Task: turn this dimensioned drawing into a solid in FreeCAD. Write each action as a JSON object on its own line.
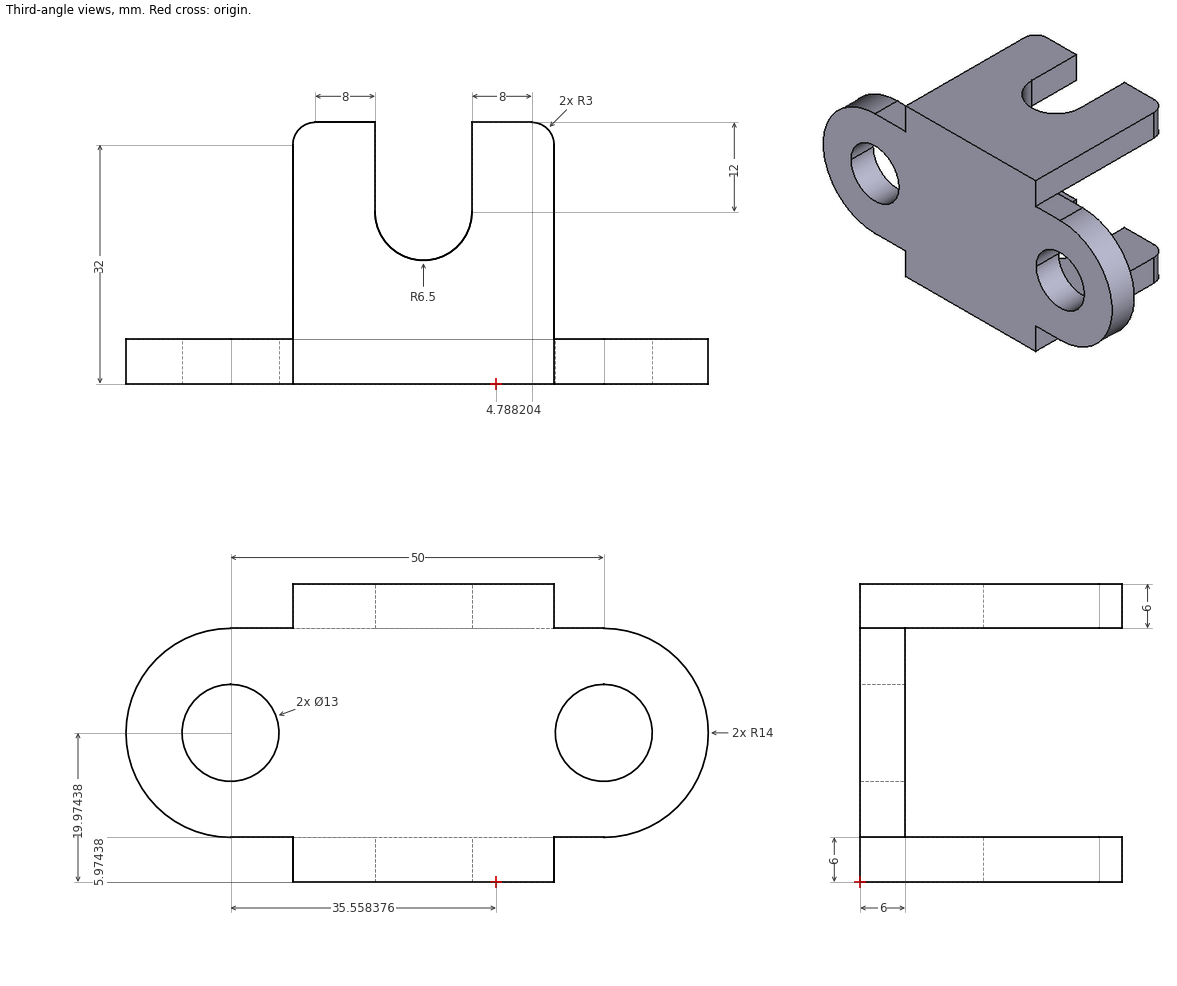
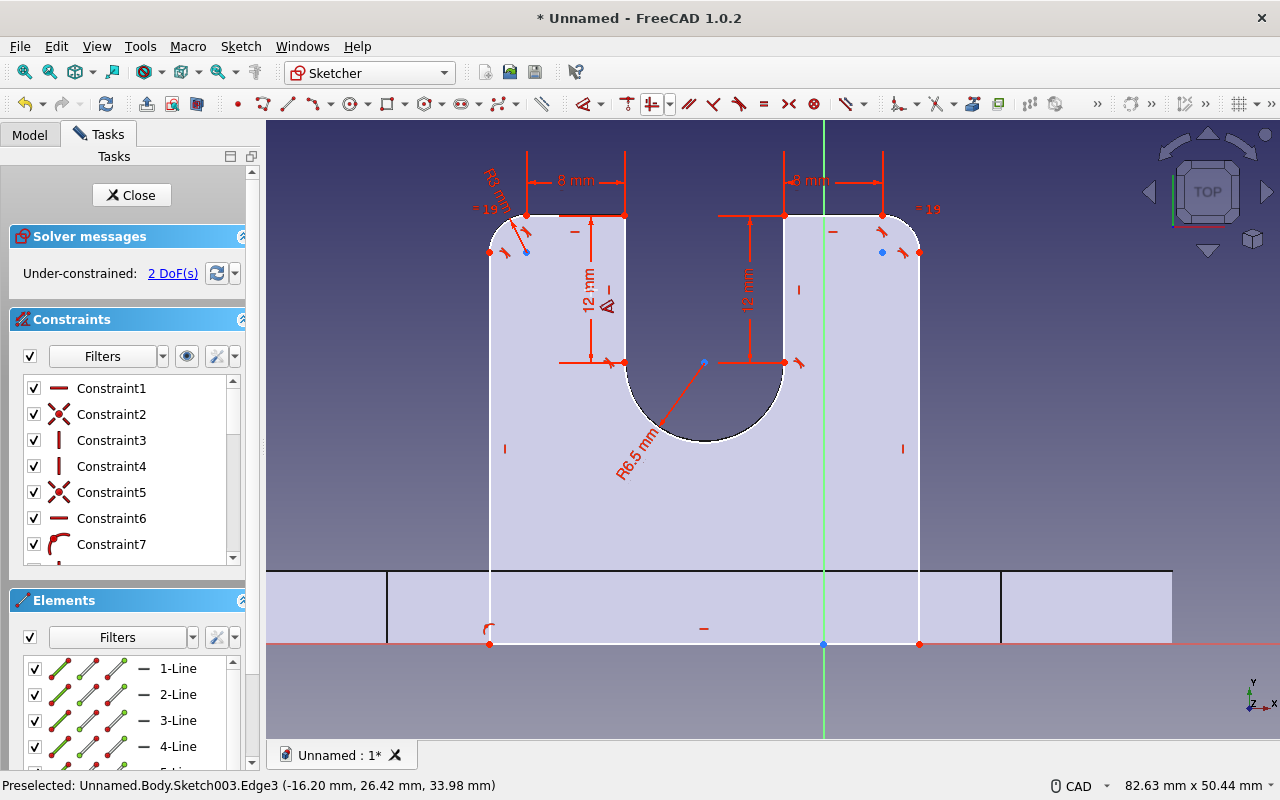
{"action": "left_click", "coordinate": [490, 370]}
{"action": "left_click", "coordinate": [456, 448]}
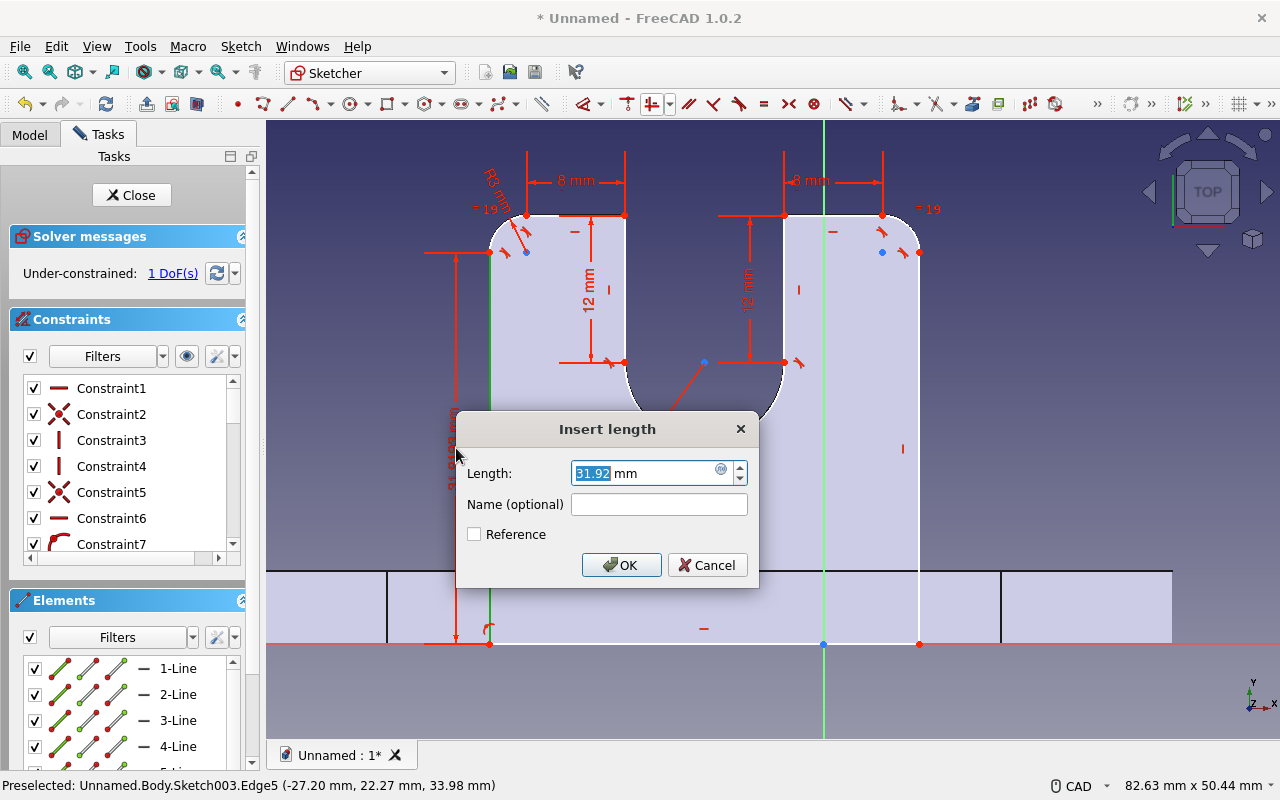
{"action": "type", "text": "32"}
{"action": "key", "text": "Return"}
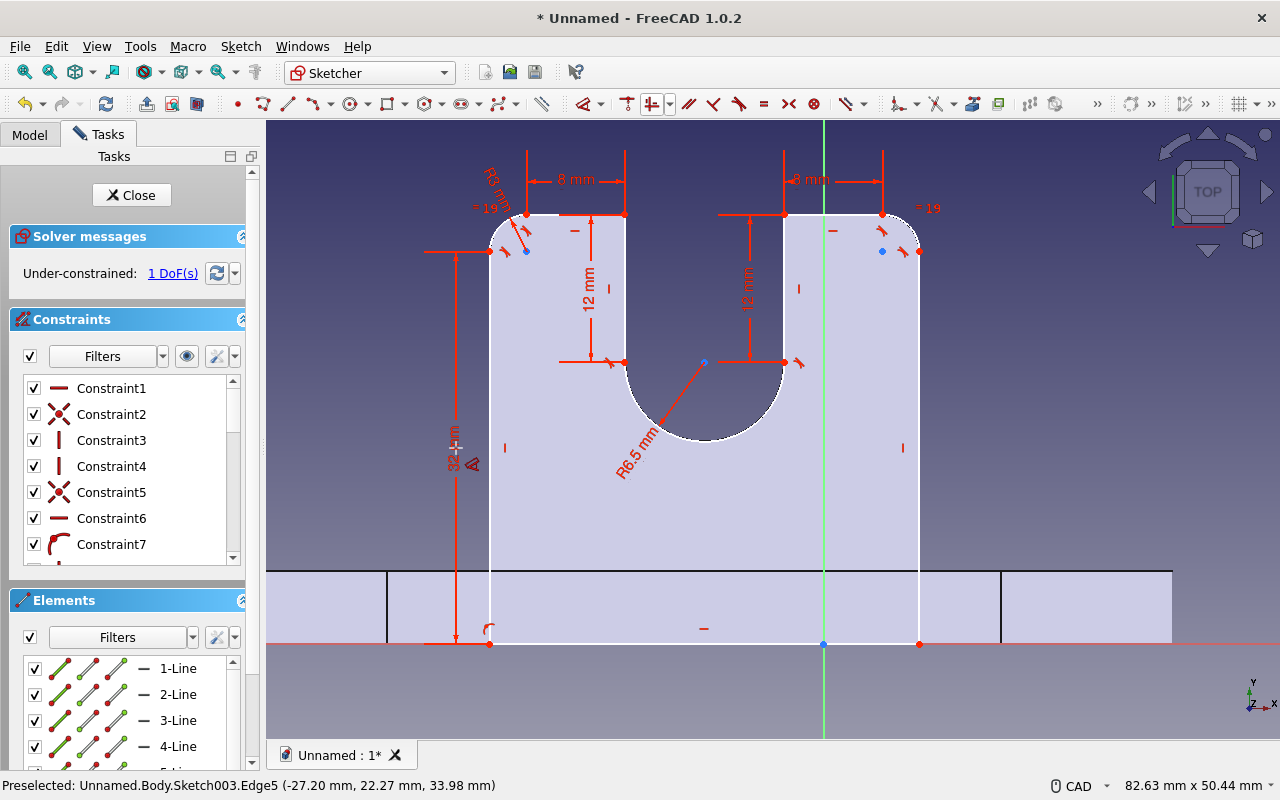
{"action": "left_click", "coordinate": [883, 215]}
{"action": "left_click", "coordinate": [853, 678]}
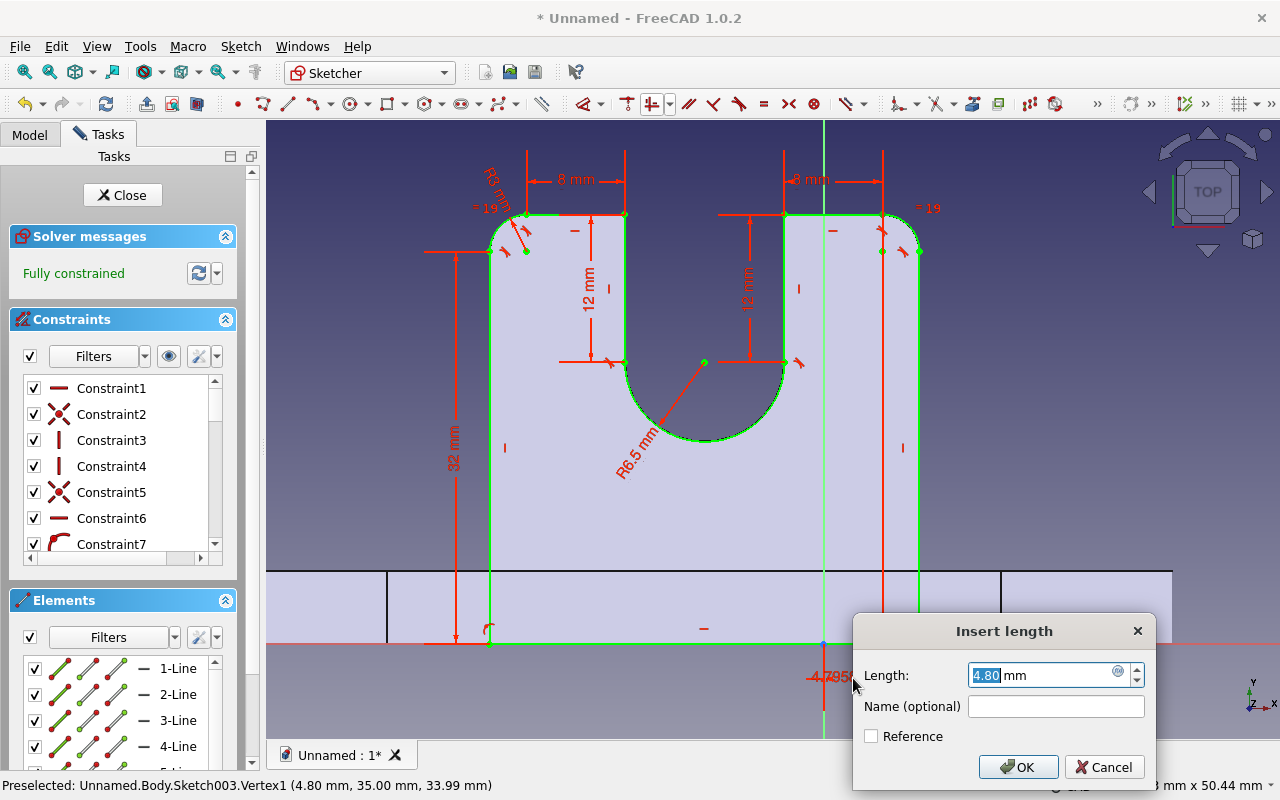
{"action": "type", "text": "4.788204"}
{"action": "key", "text": "Return"}
{"action": "key", "text": "Escape"}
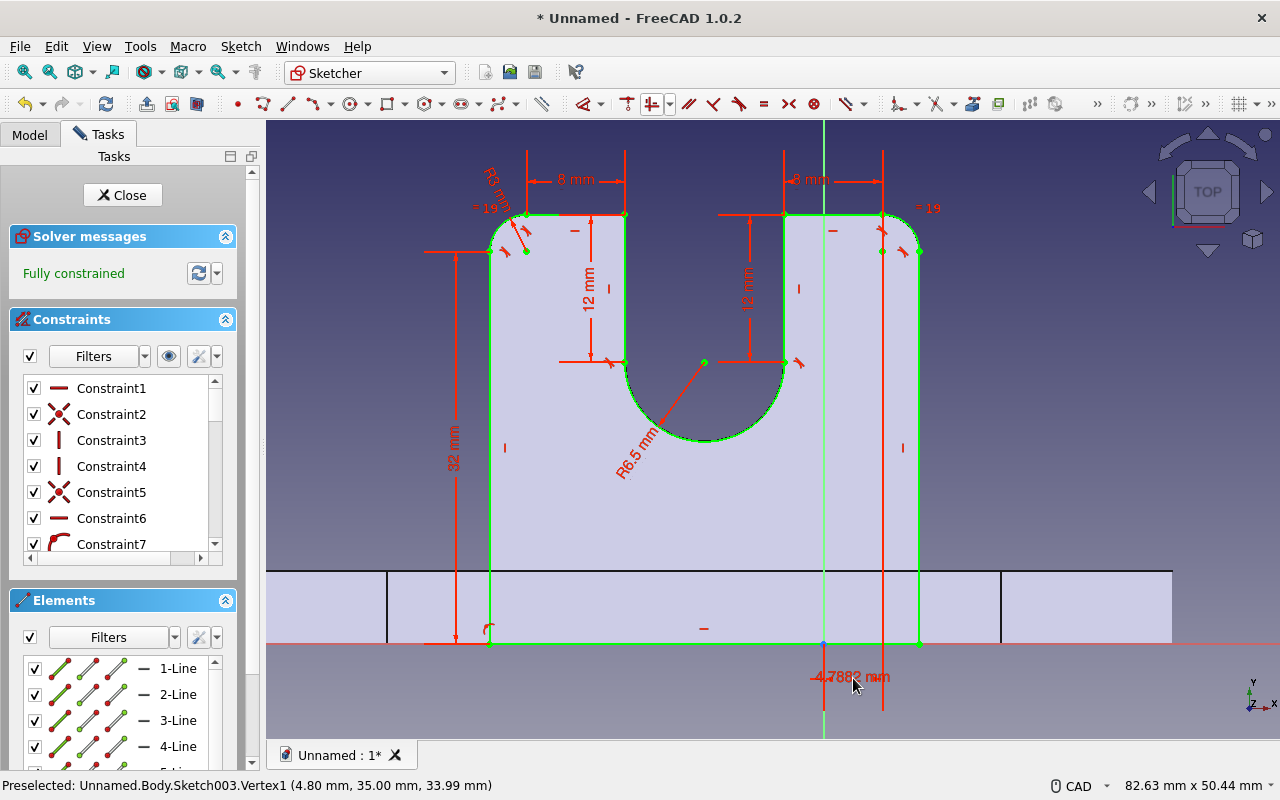
{"action": "left_click", "coordinate": [123, 195]}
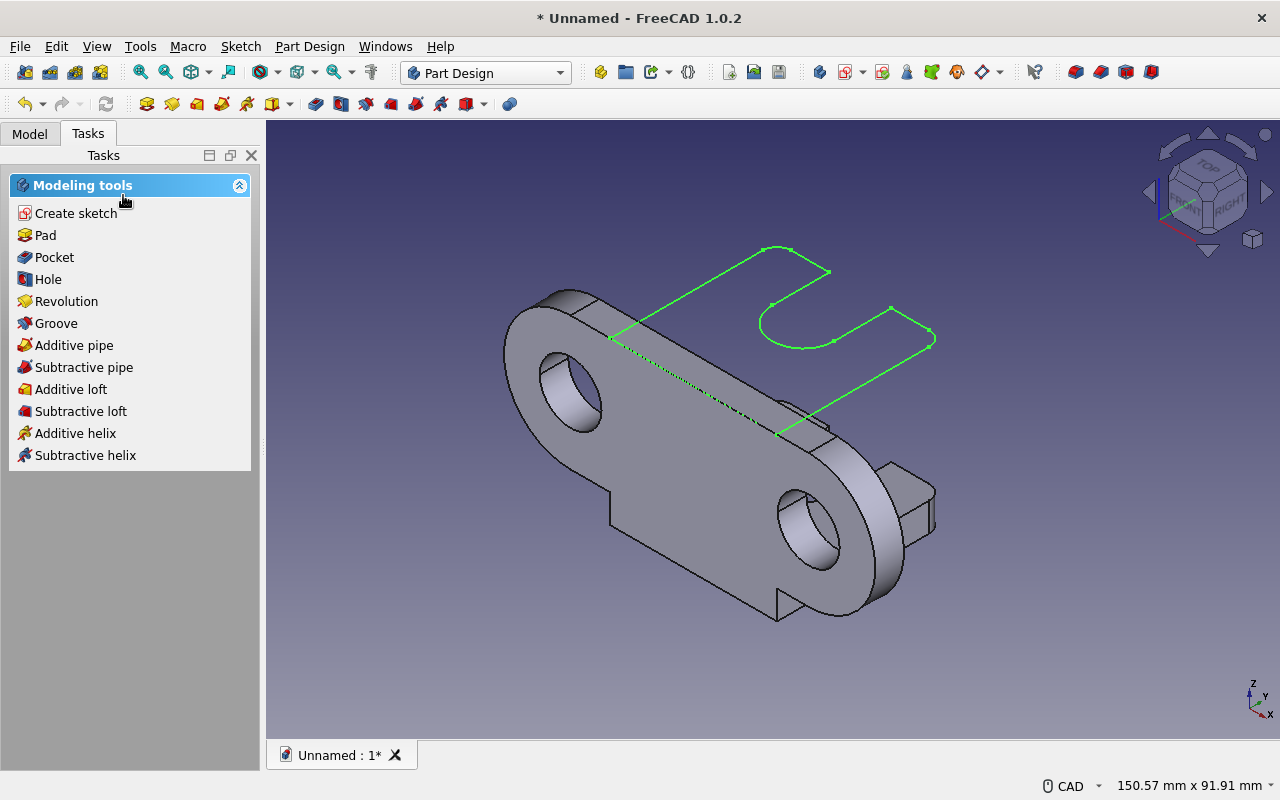
{"action": "left_click", "coordinate": [147, 104]}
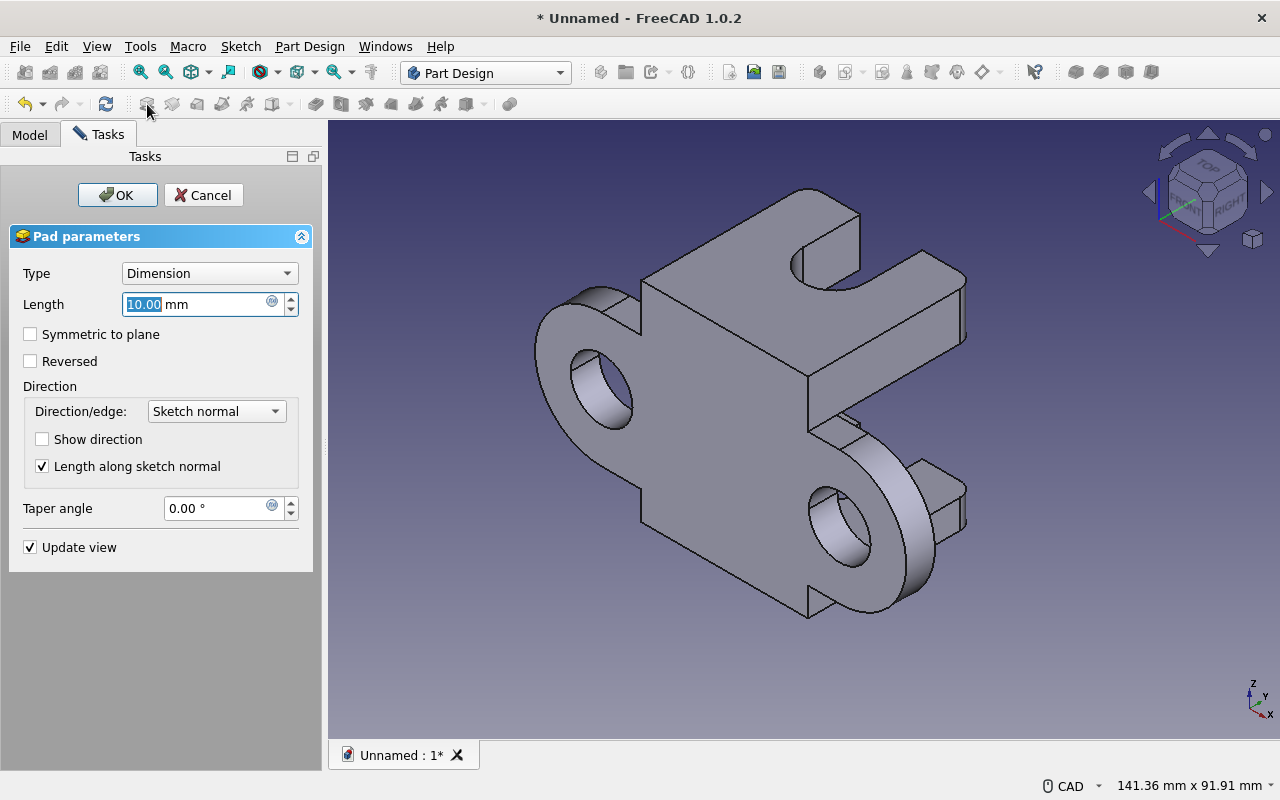
{"action": "type", "text": "6"}
{"action": "key", "text": "Tab"}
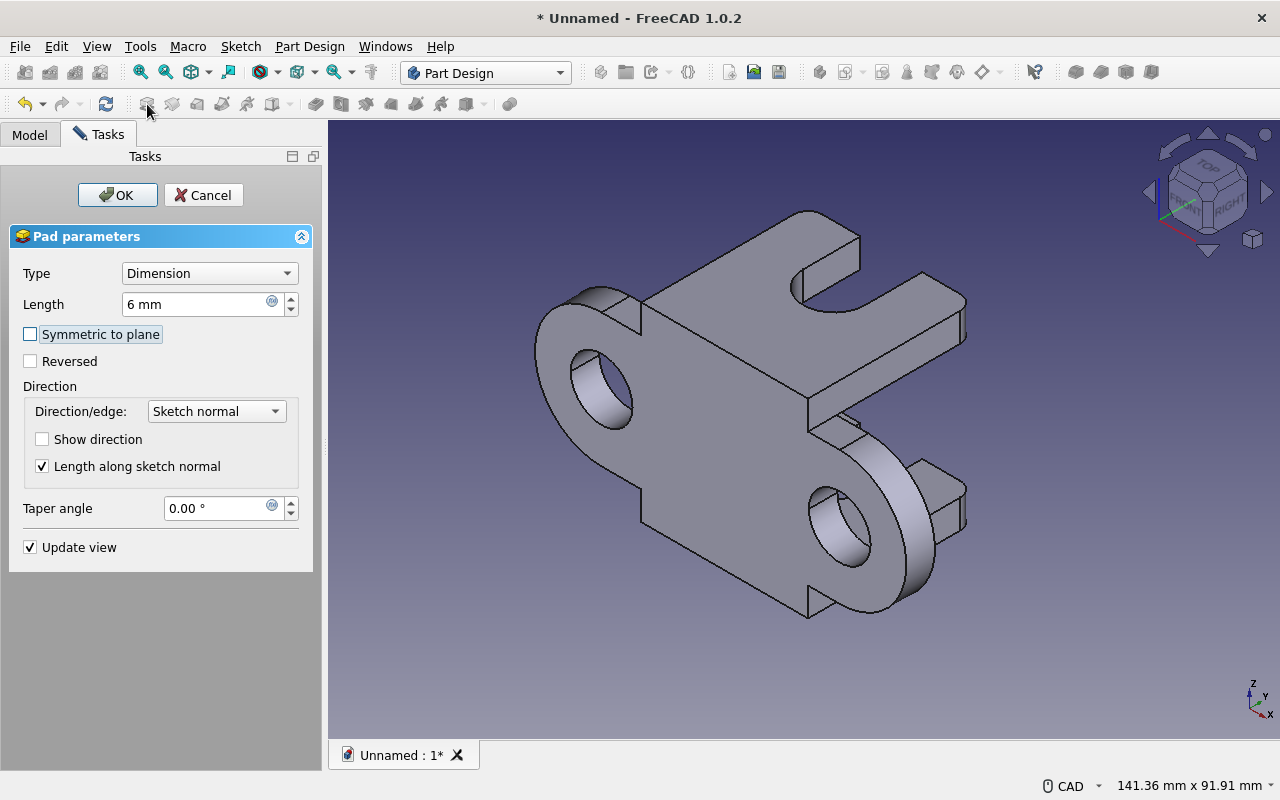
{"action": "left_click", "coordinate": [118, 195]}